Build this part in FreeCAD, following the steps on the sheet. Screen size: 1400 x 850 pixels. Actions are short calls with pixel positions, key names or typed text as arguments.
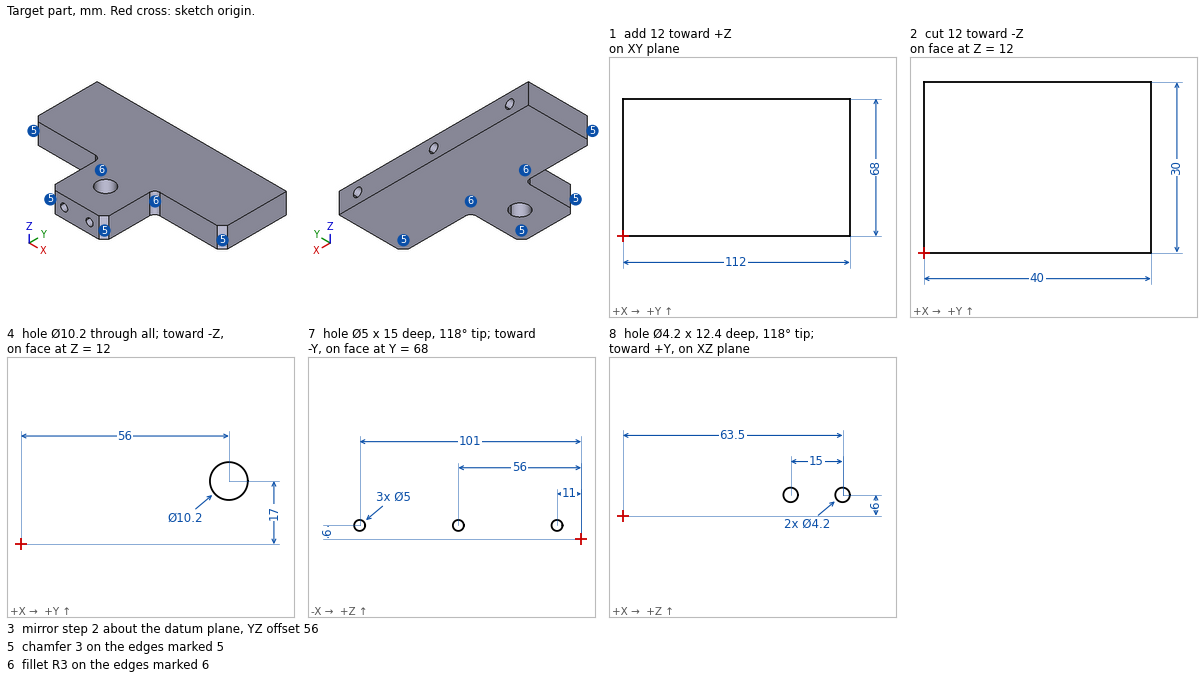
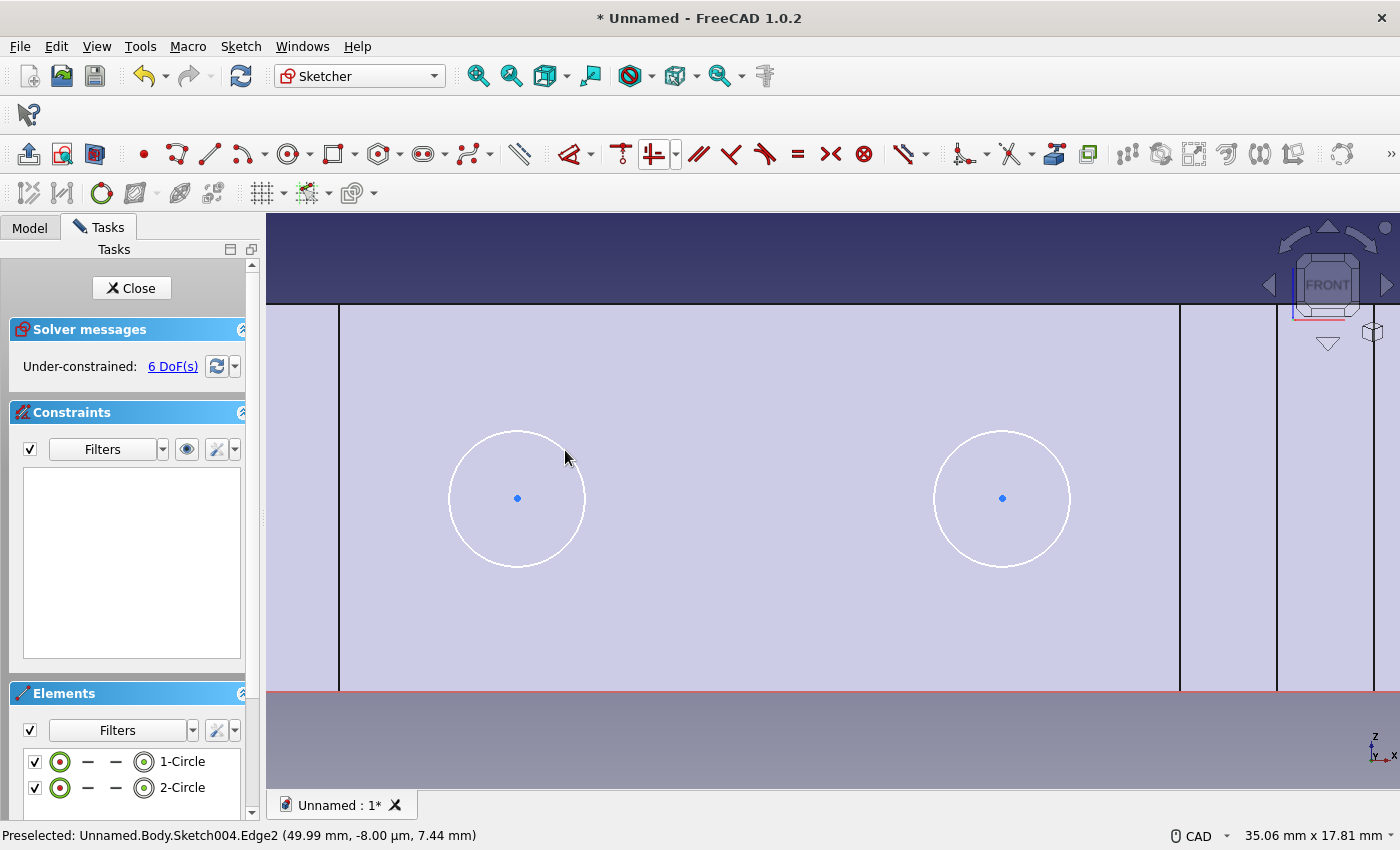
click(1050, 451)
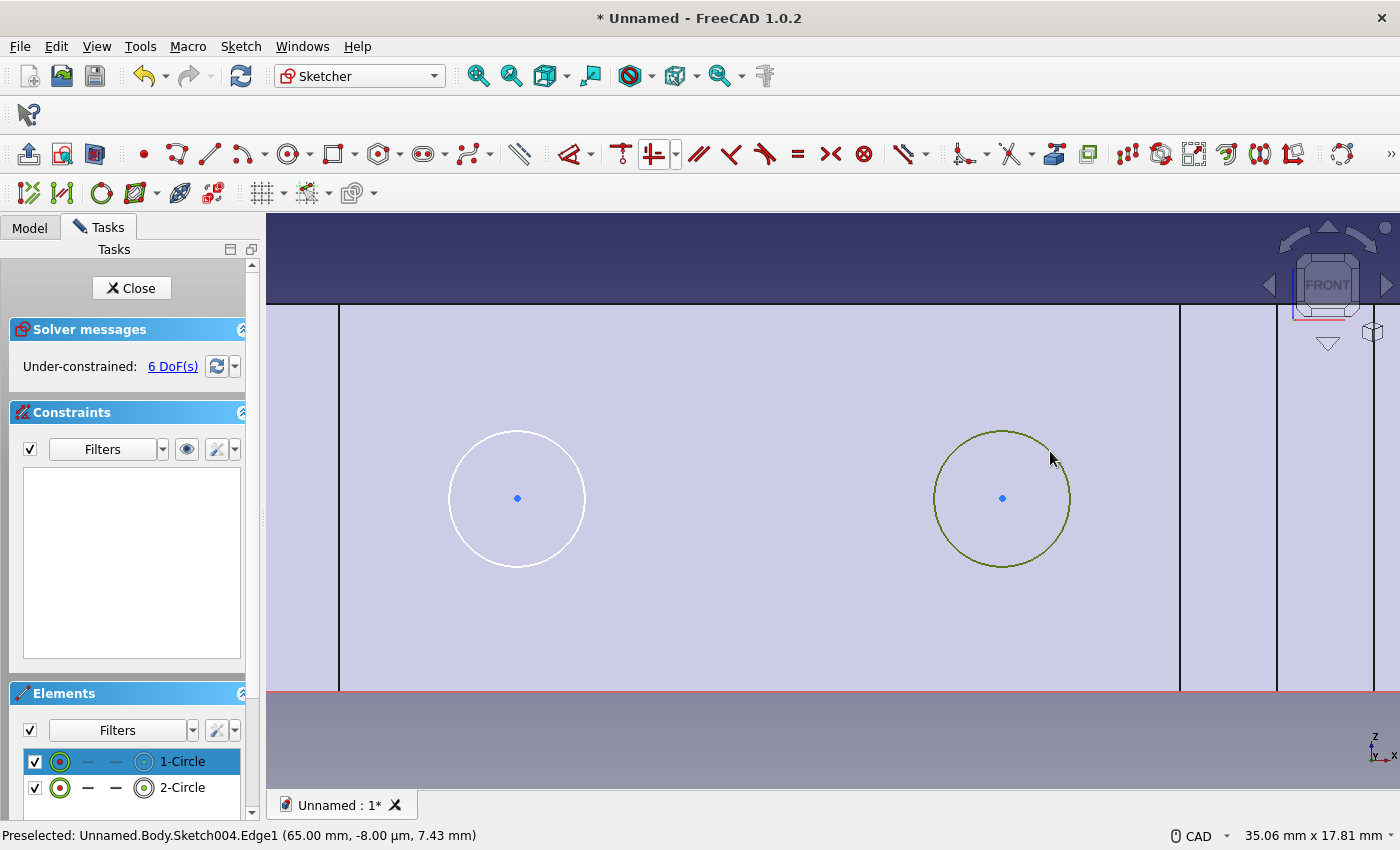
click(565, 451)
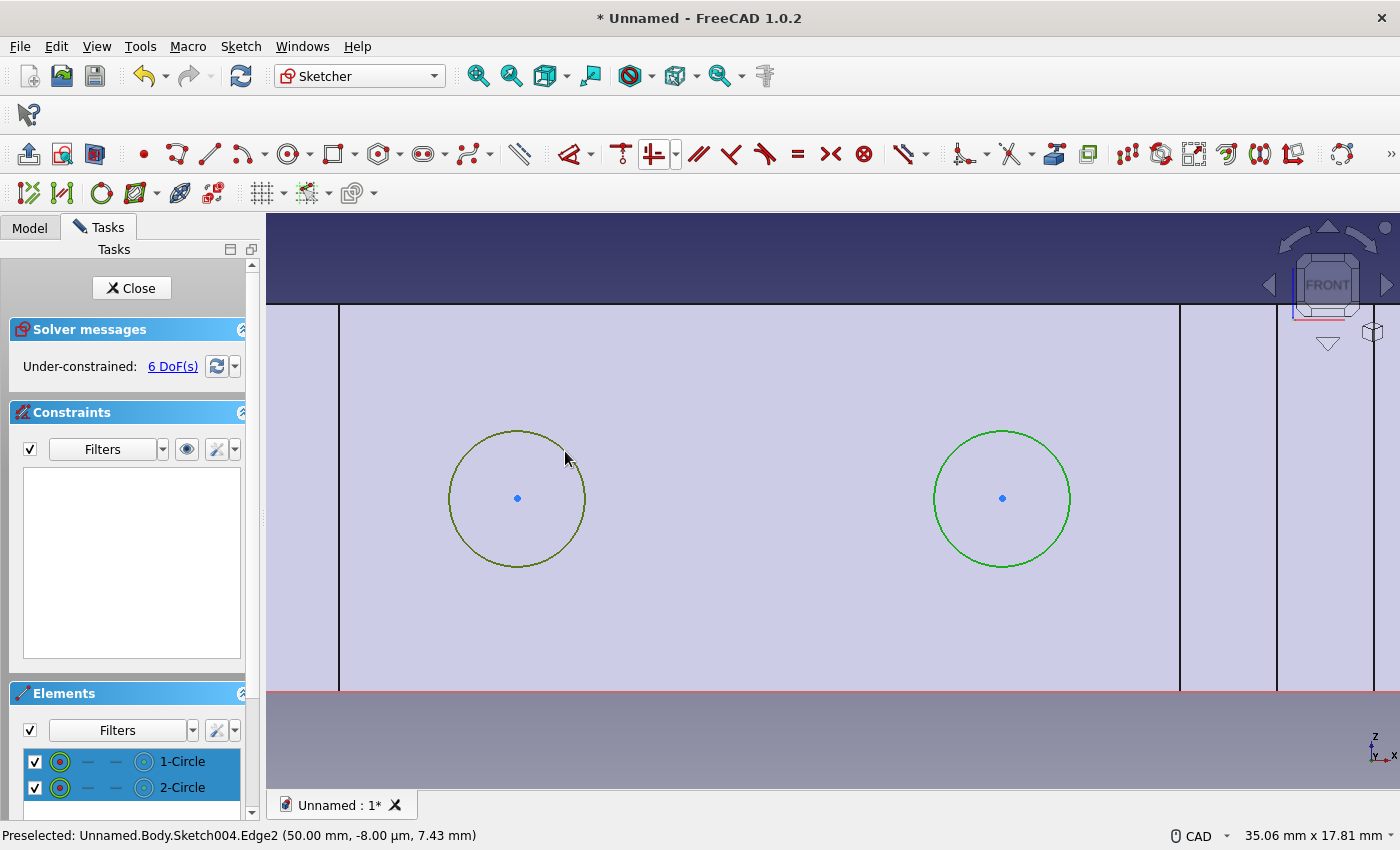
click(798, 154)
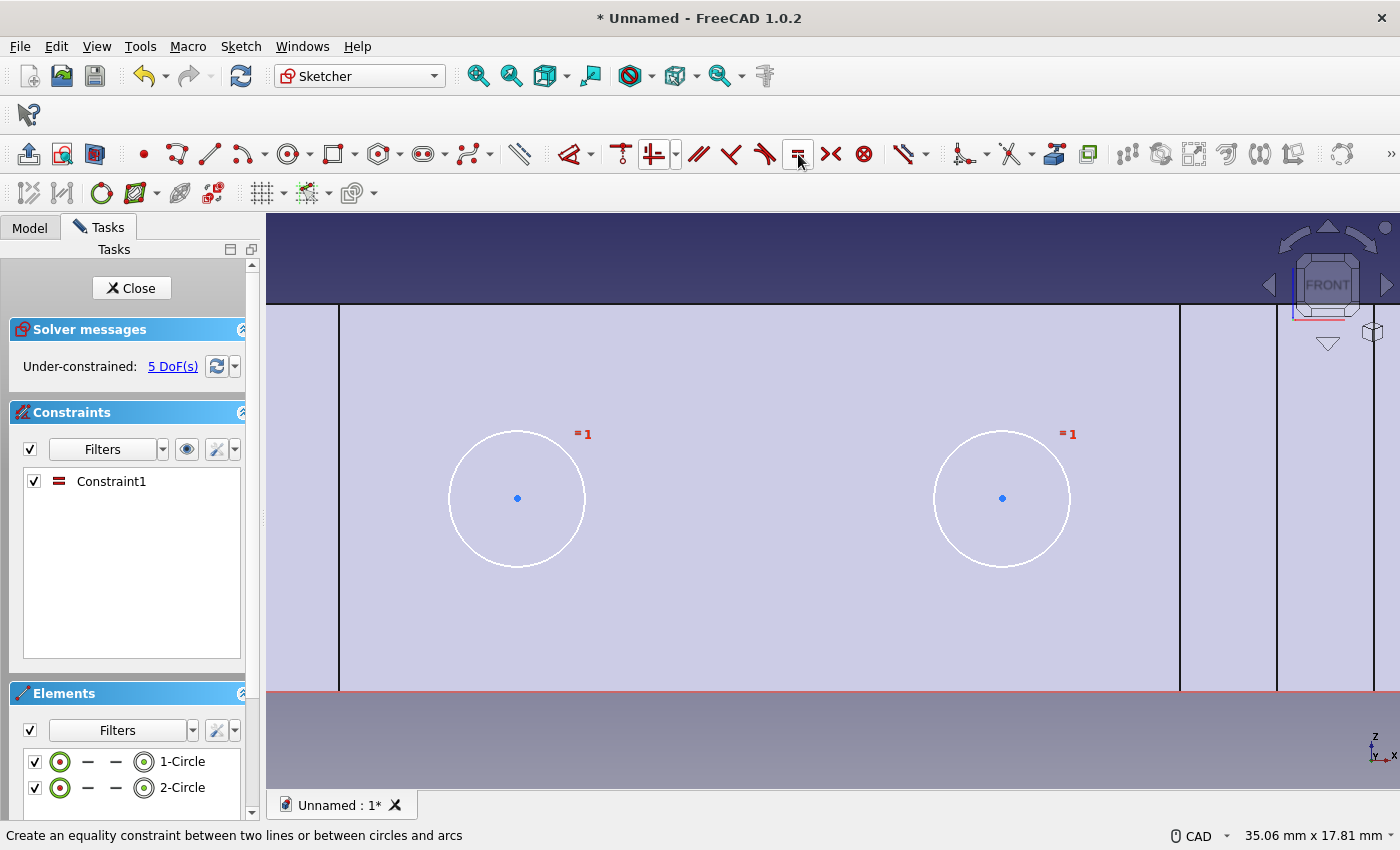
click(1002, 499)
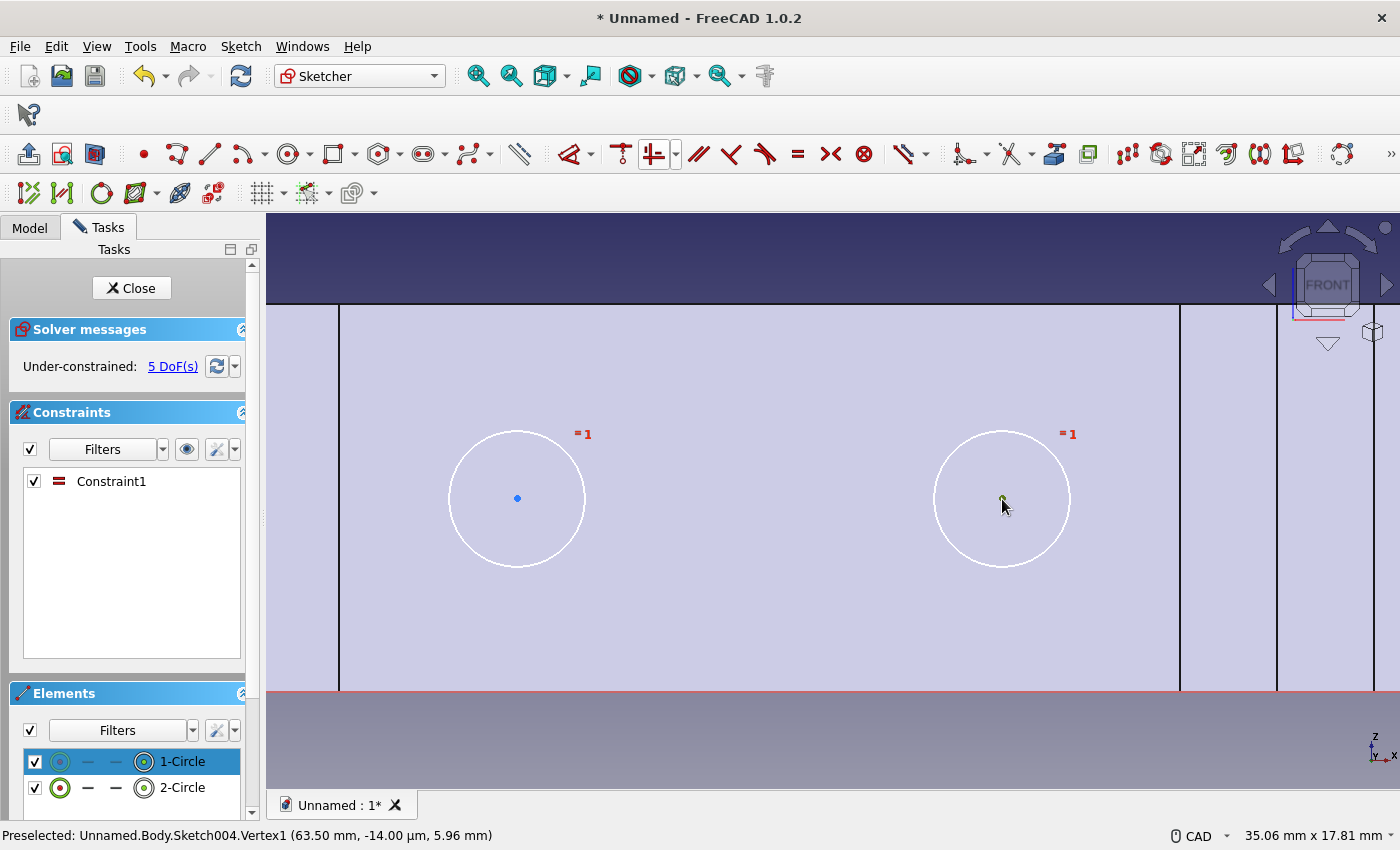
click(517, 499)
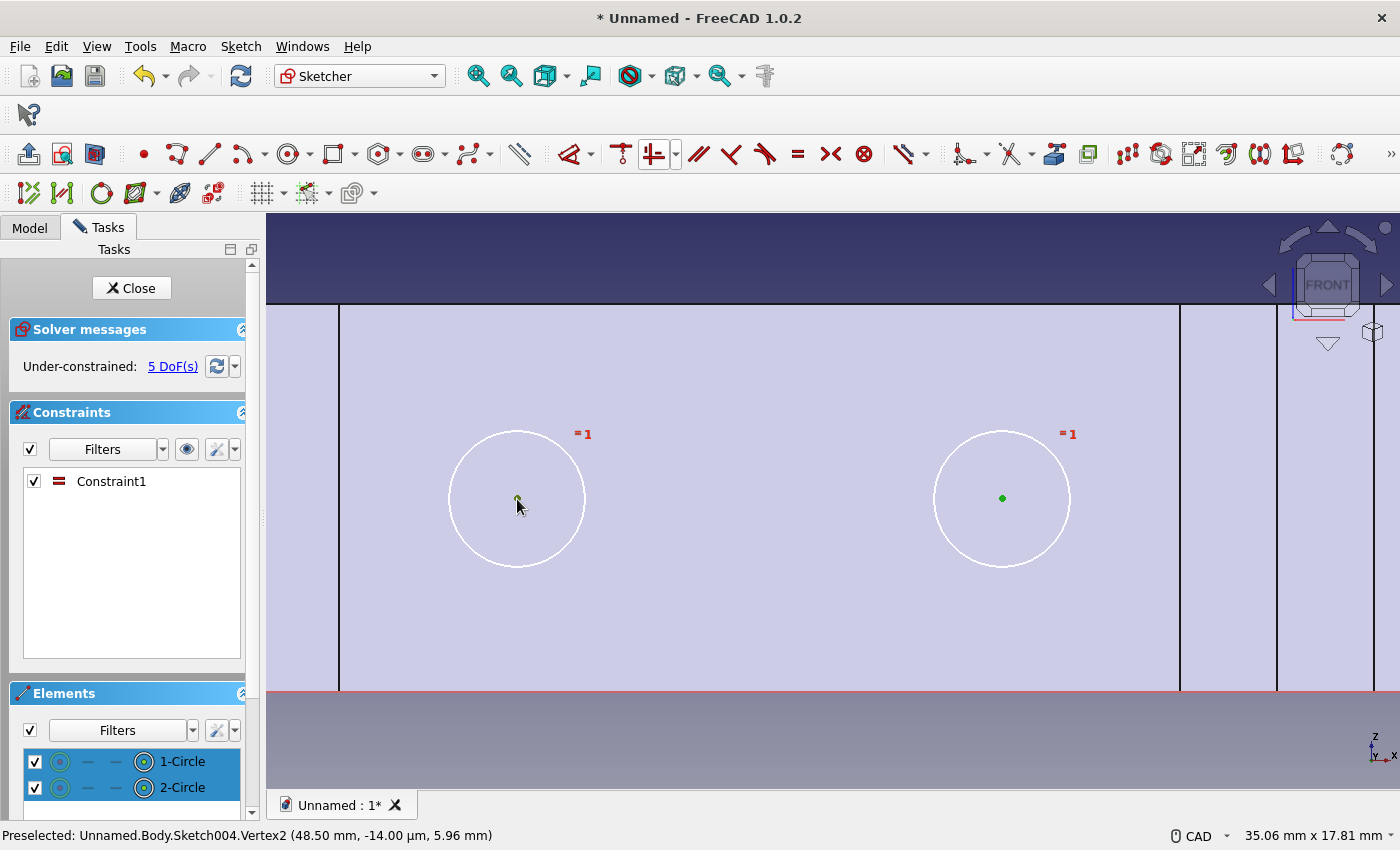
key(h)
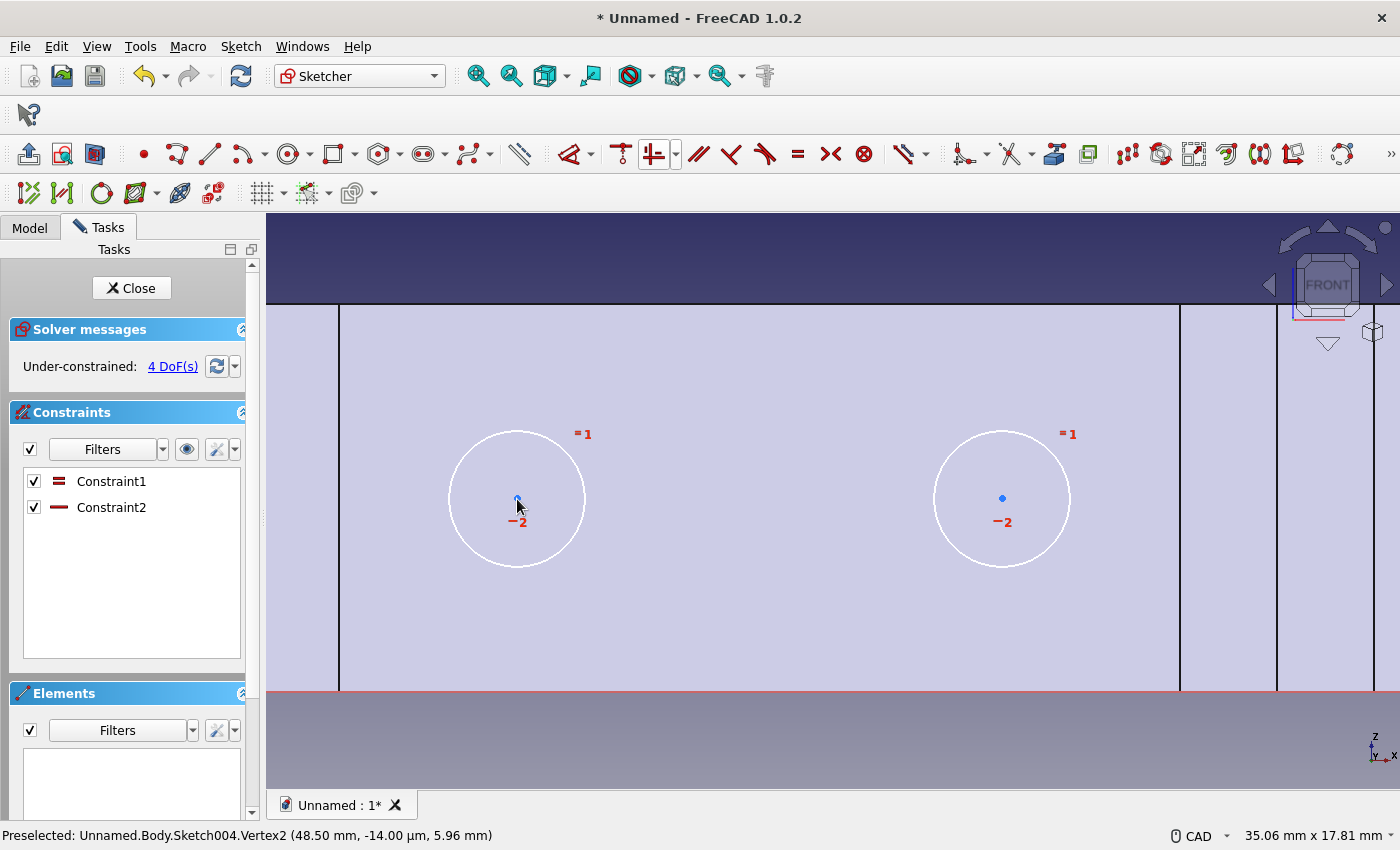
click(568, 154)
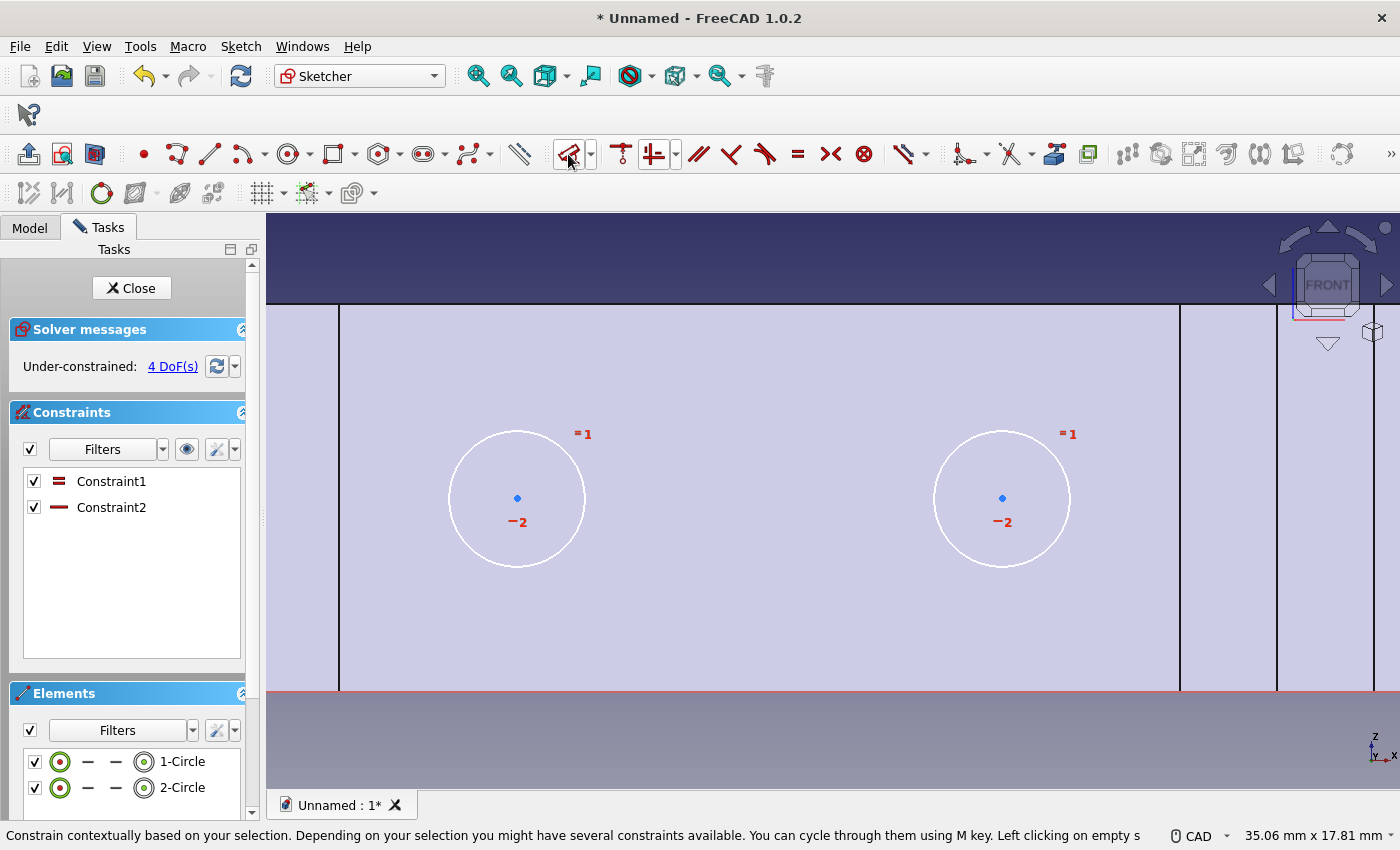
click(1050, 451)
click(1073, 428)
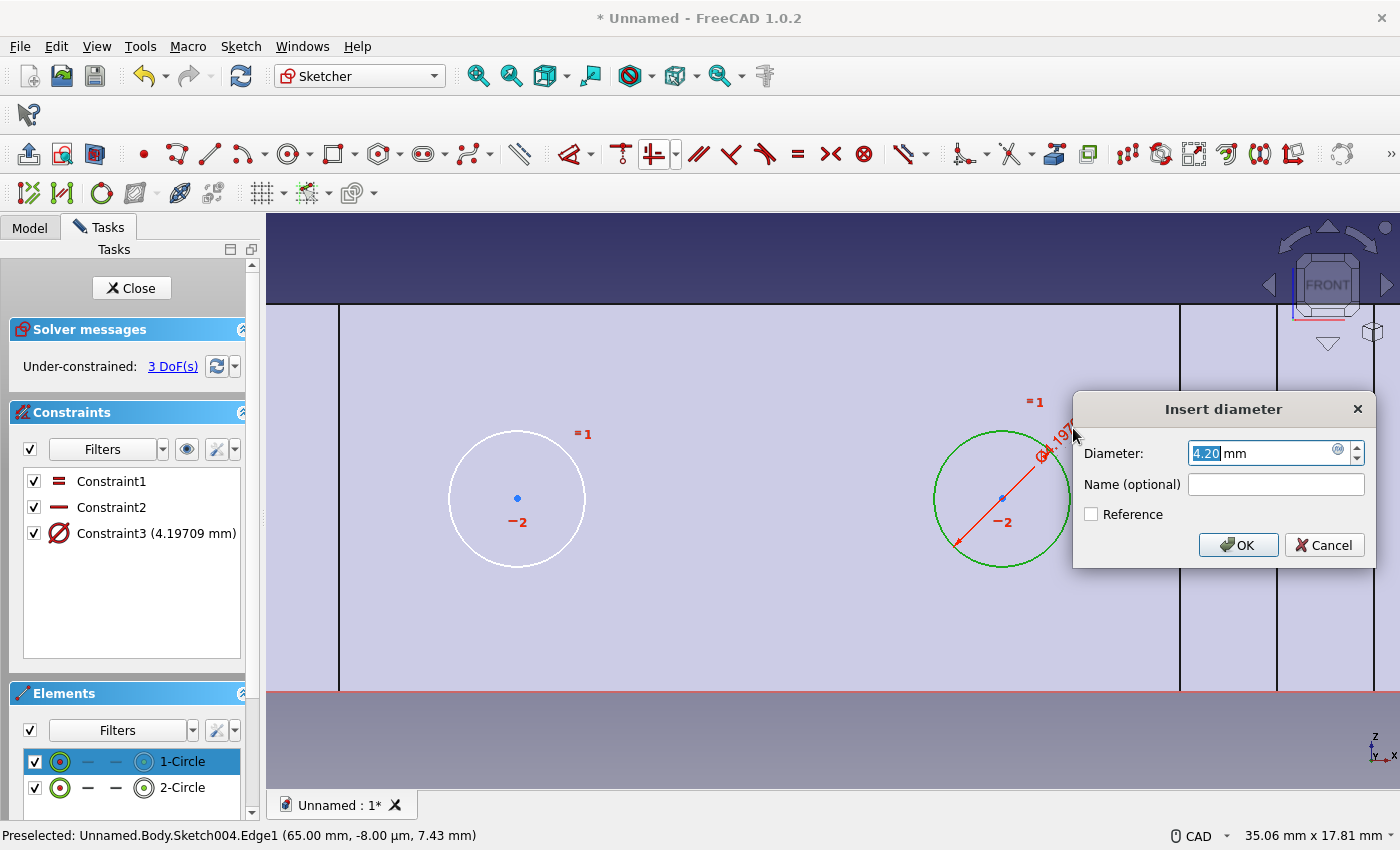
text(4.2)
key(Return)